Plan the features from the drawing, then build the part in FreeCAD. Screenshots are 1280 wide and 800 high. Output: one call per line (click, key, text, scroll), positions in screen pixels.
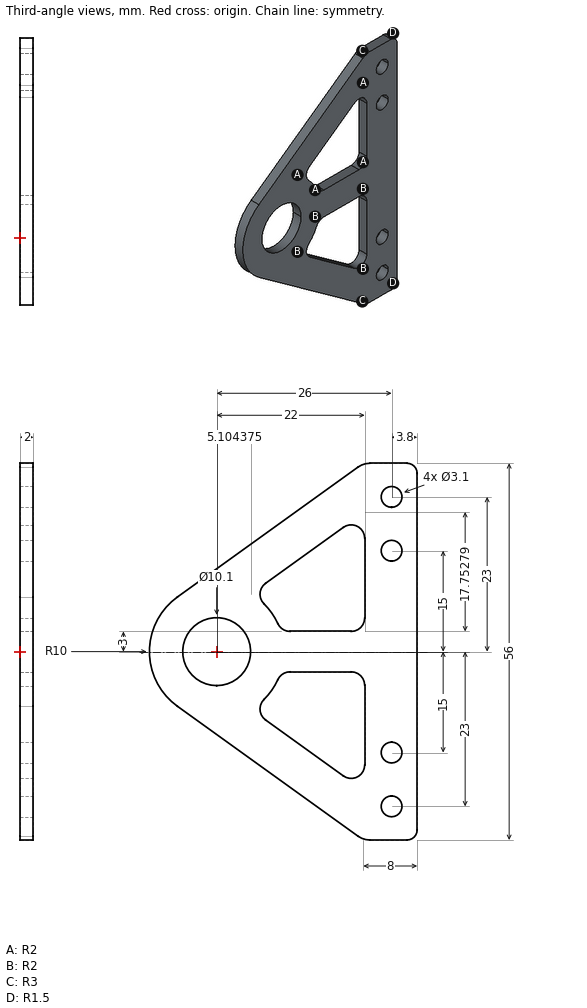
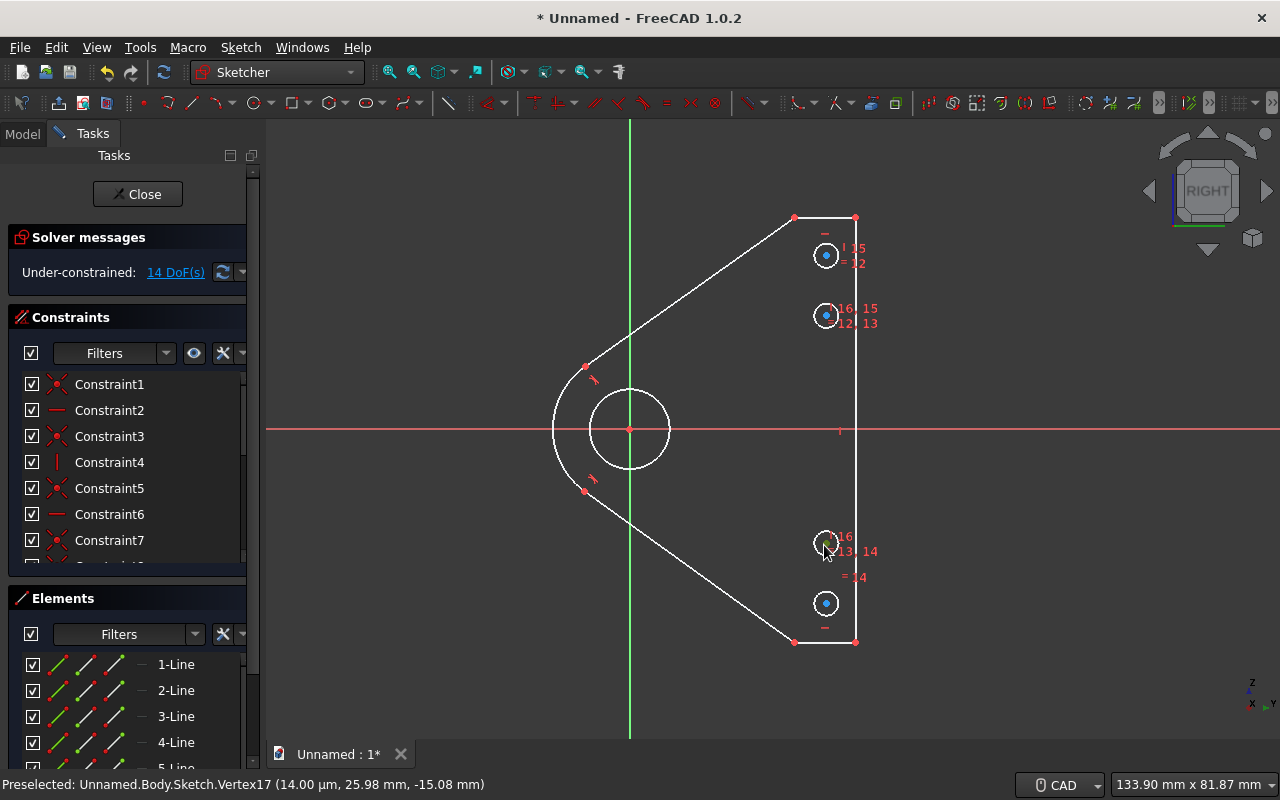
click(826, 604)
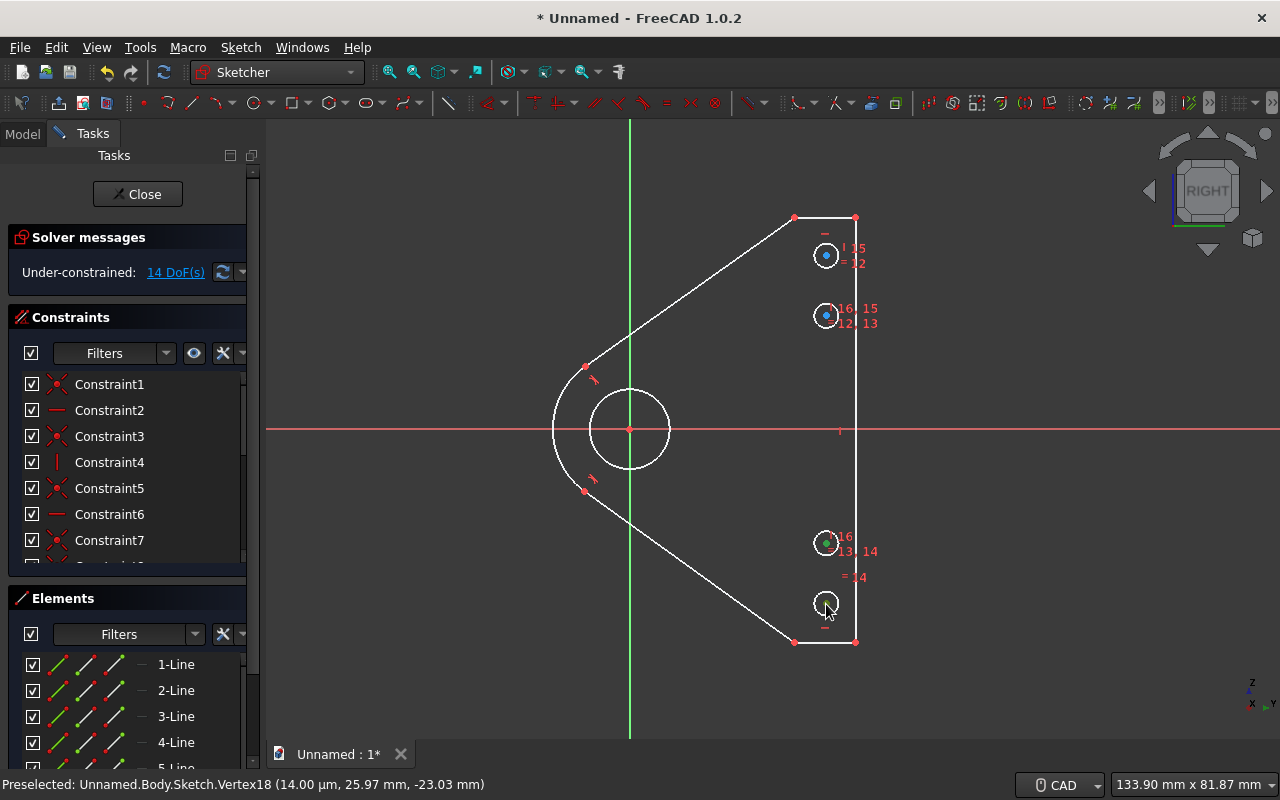
key(v)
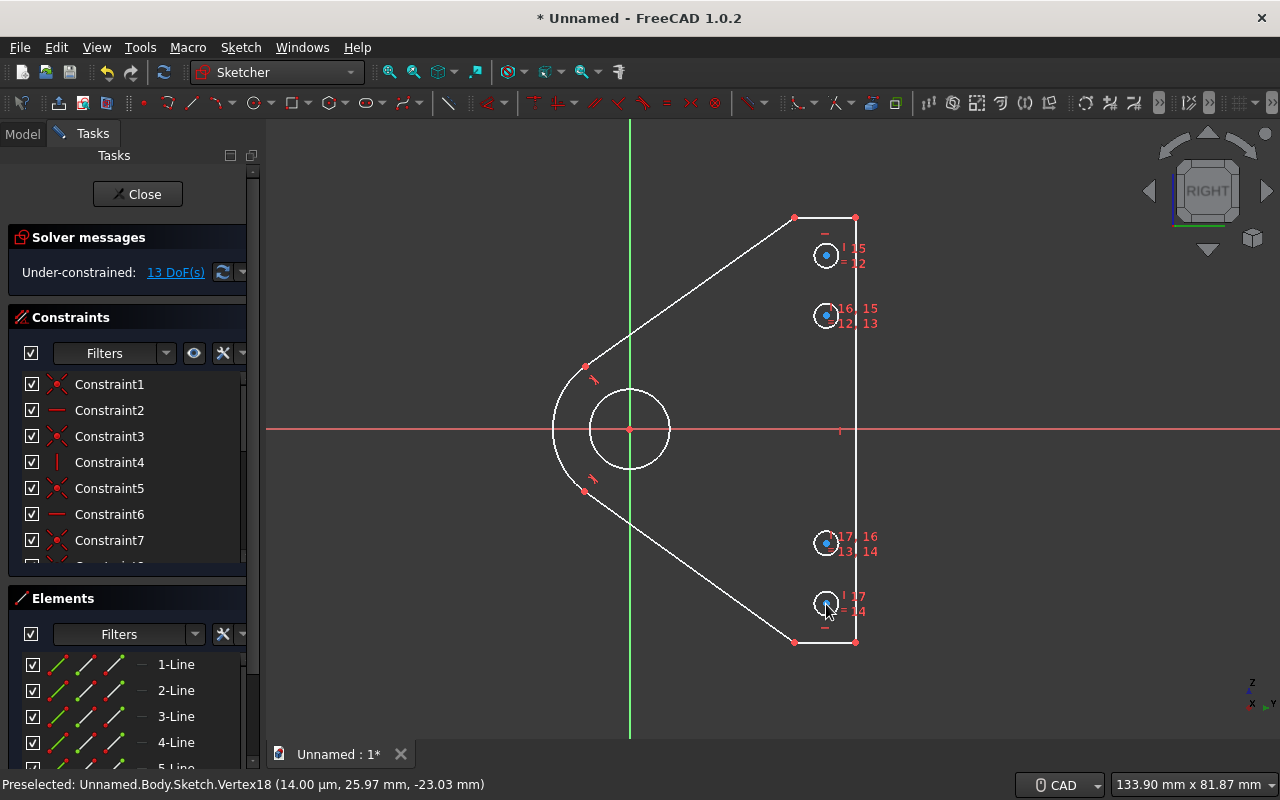
click(795, 643)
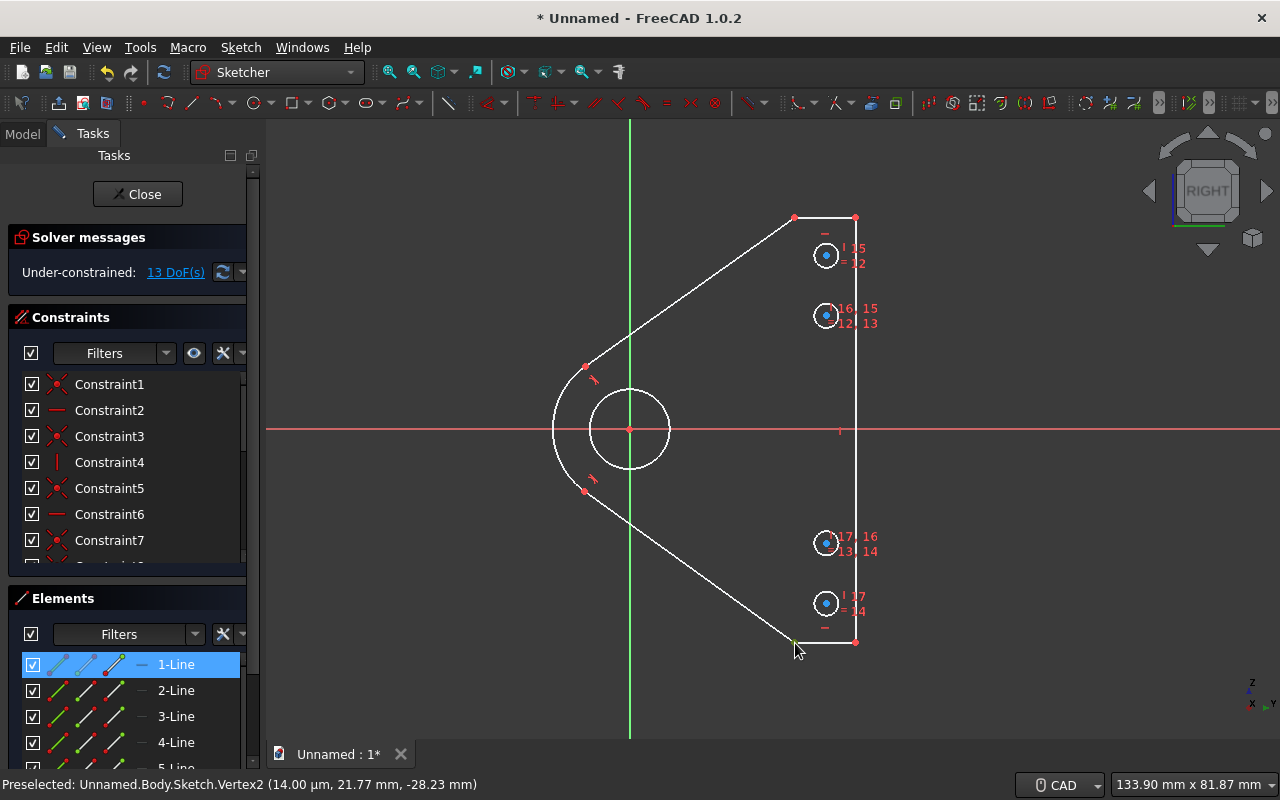
click(795, 218)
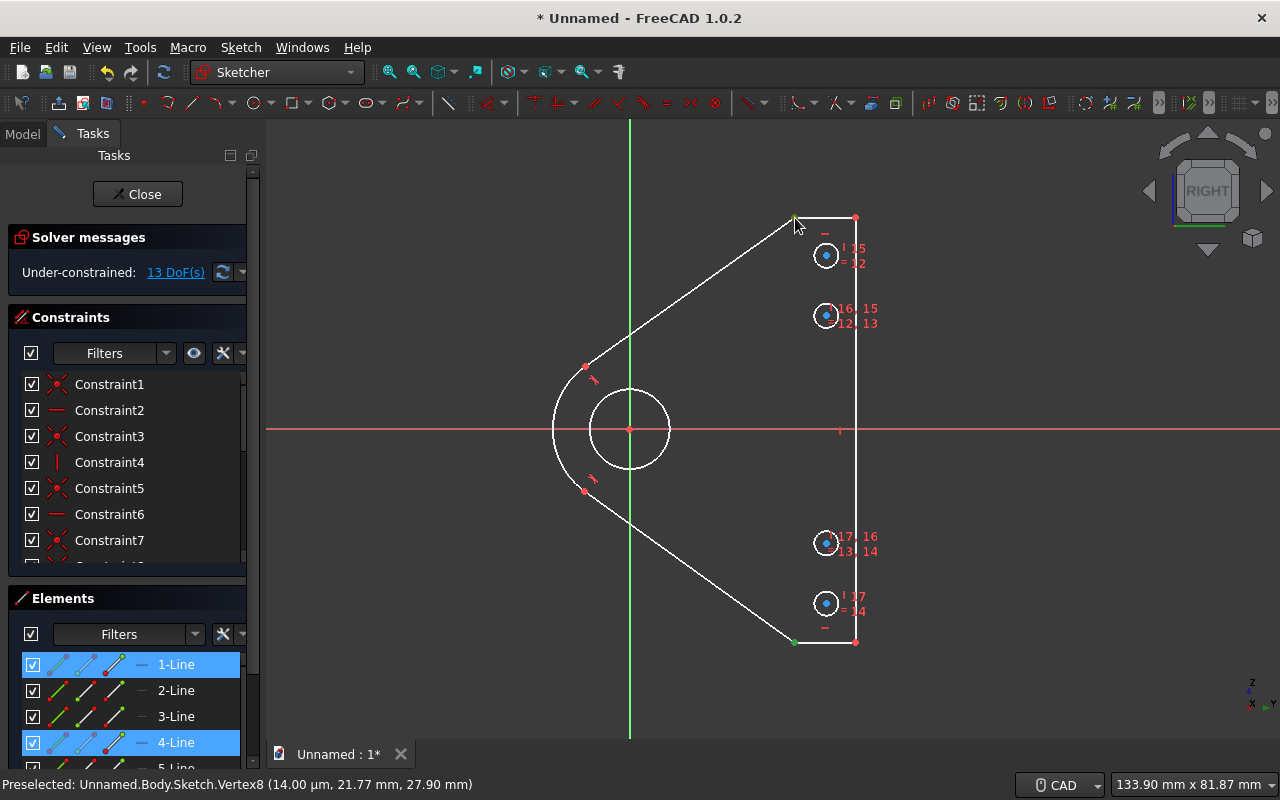
click(353, 429)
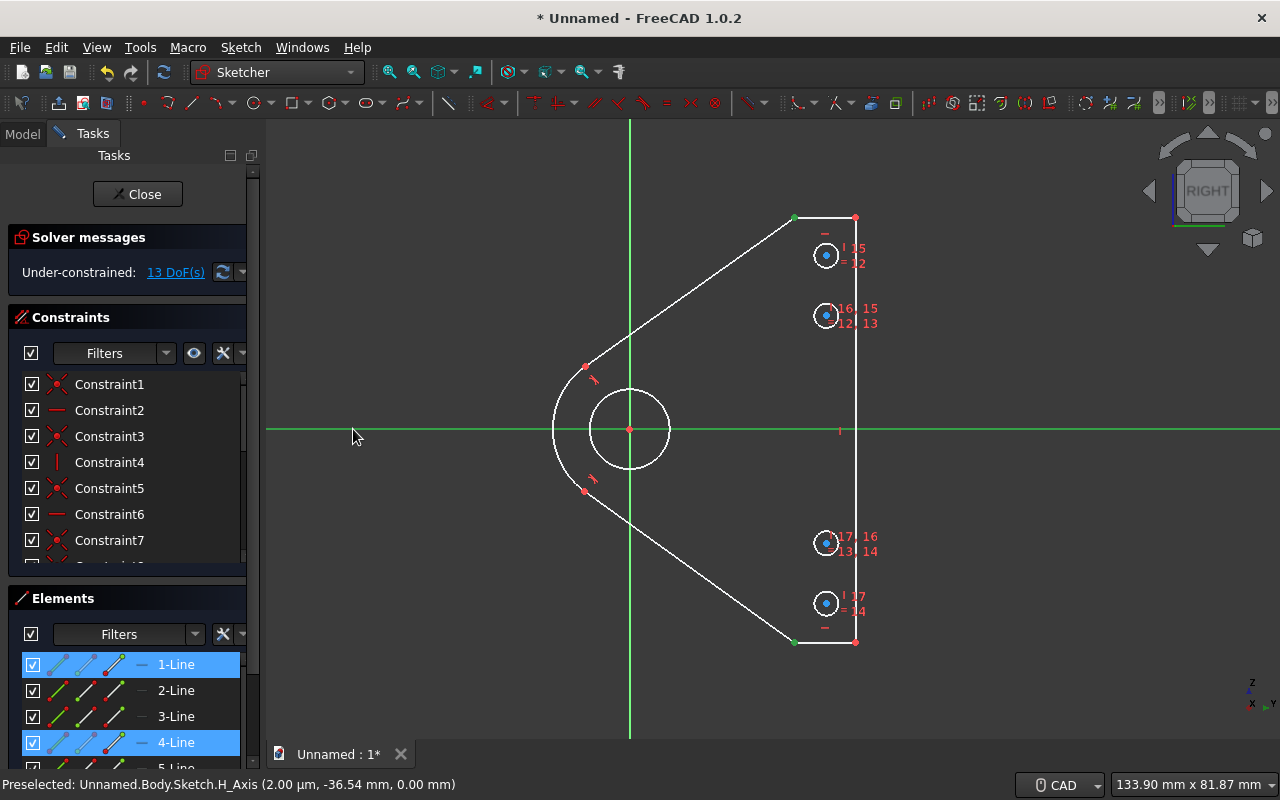
click(692, 104)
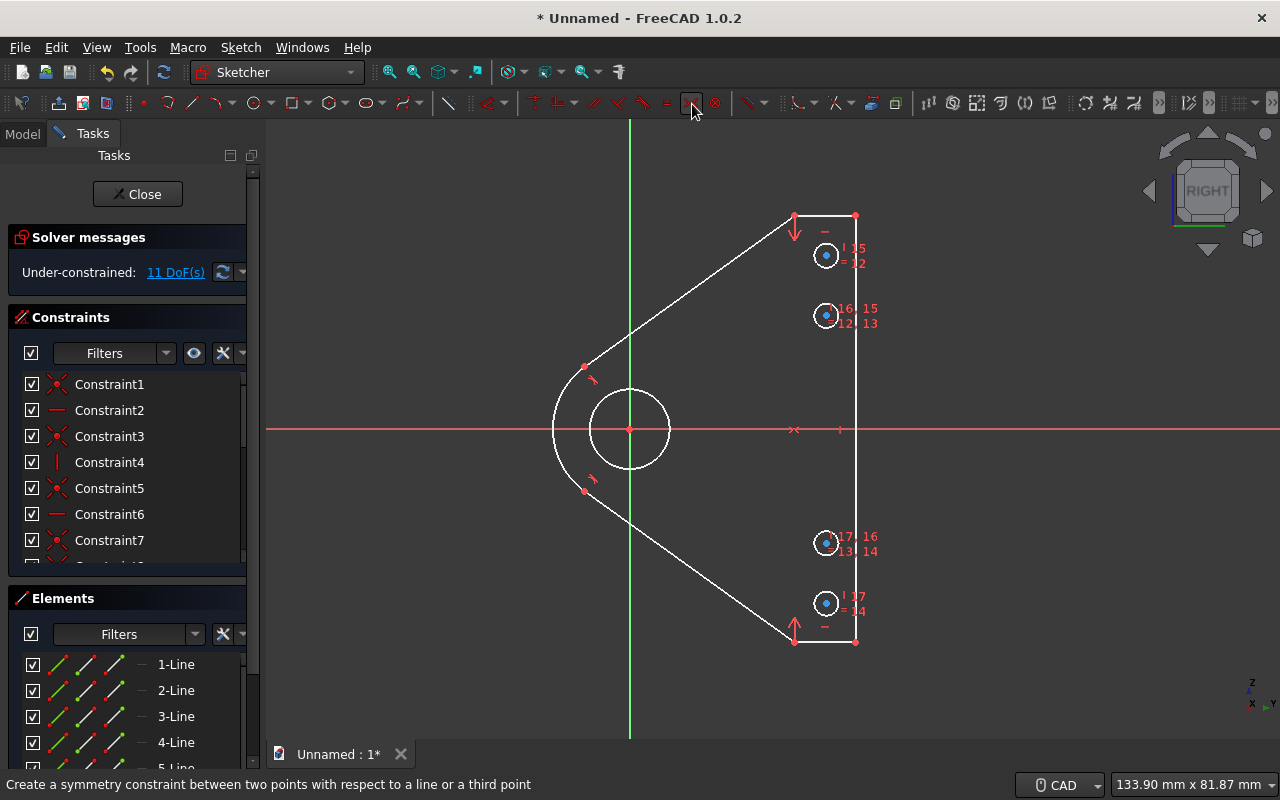
click(488, 104)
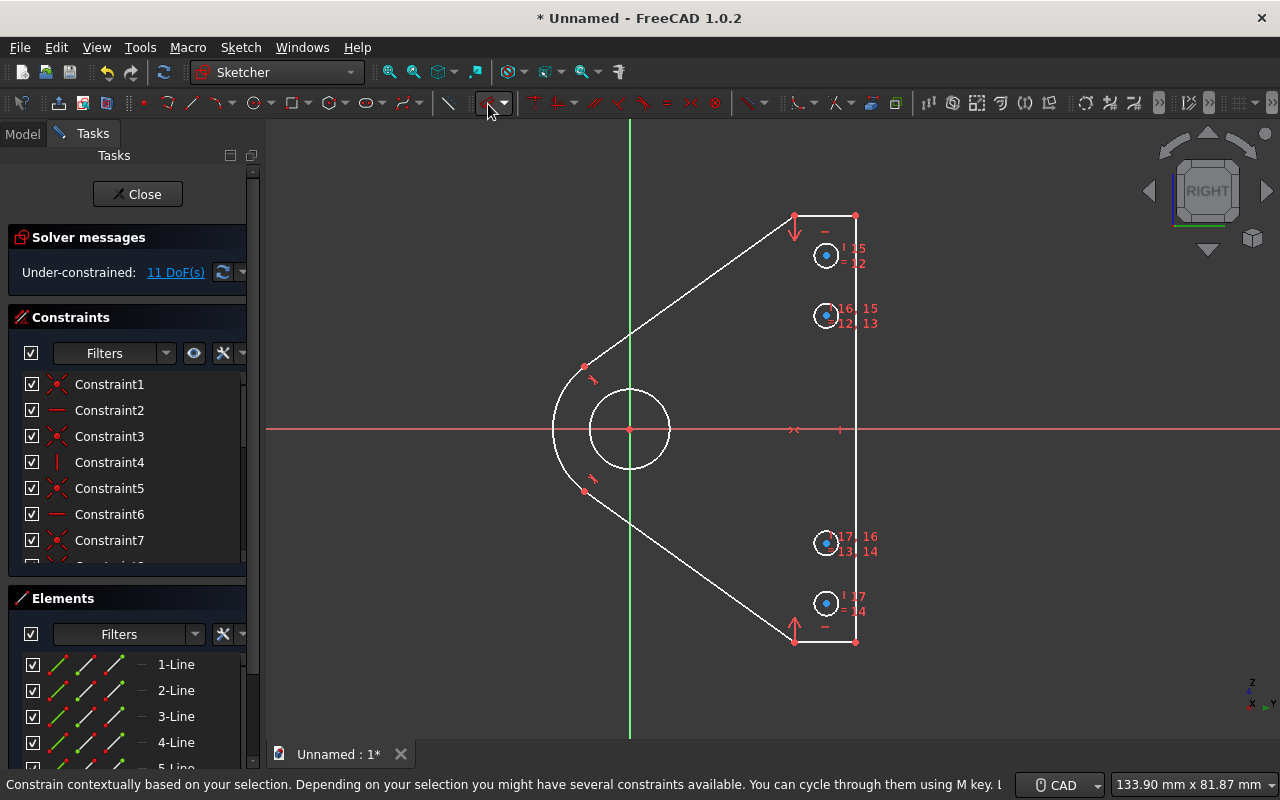
click(558, 401)
click(528, 389)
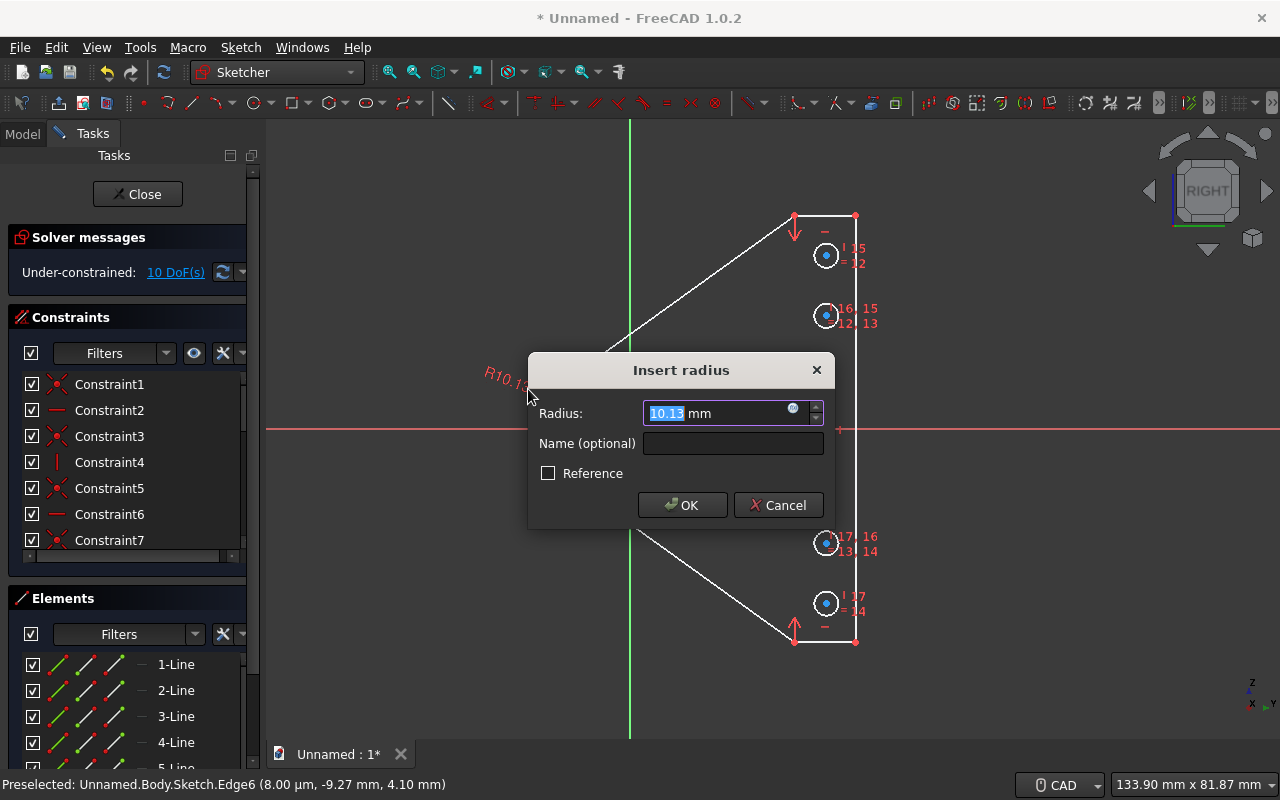
text(10)
key(Return)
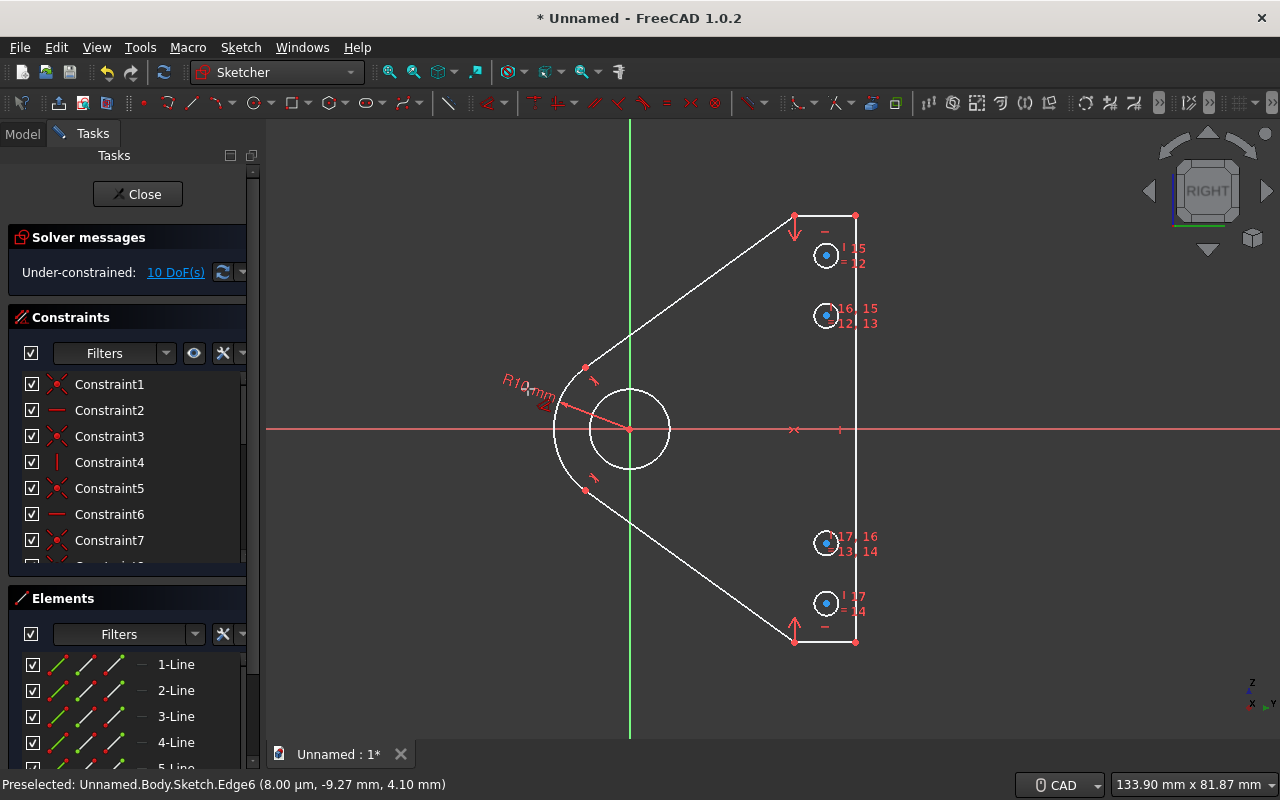
click(658, 401)
click(681, 378)